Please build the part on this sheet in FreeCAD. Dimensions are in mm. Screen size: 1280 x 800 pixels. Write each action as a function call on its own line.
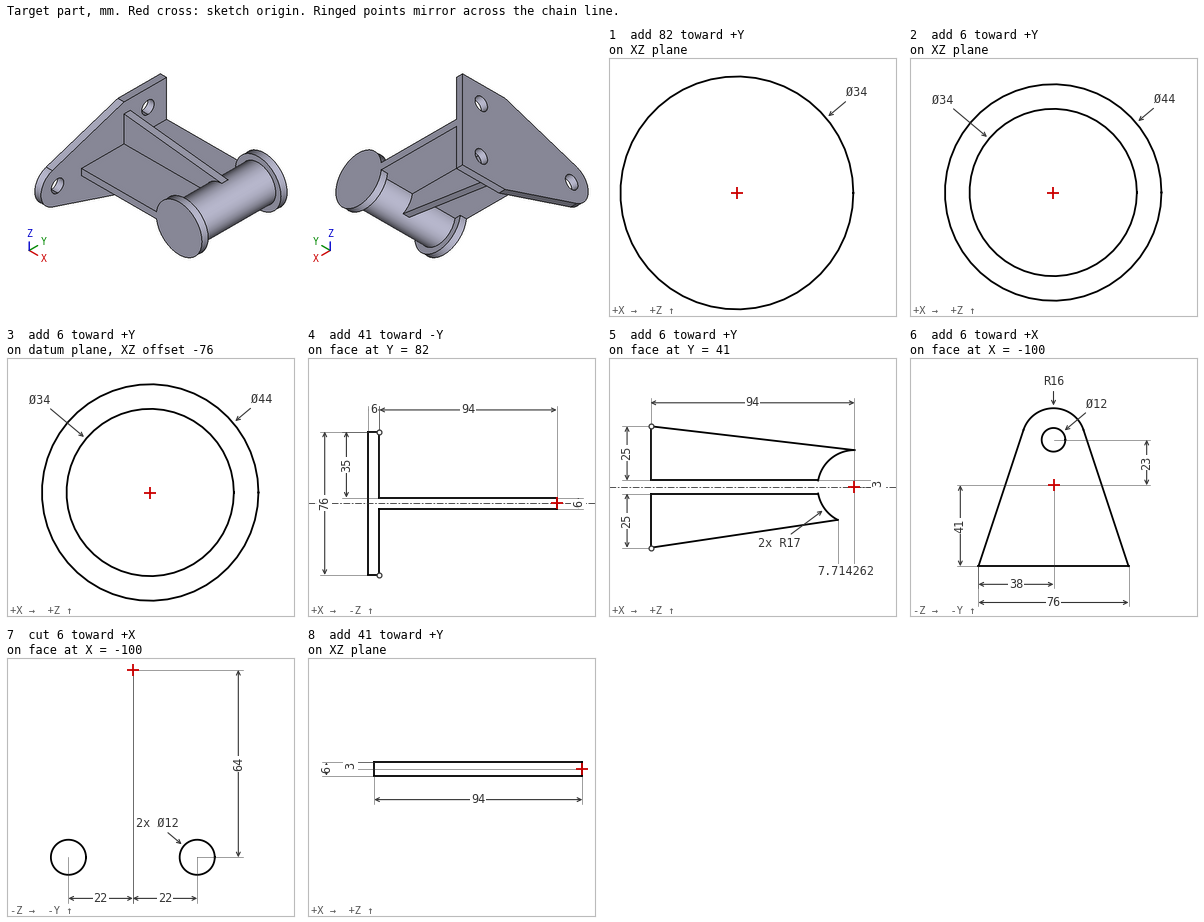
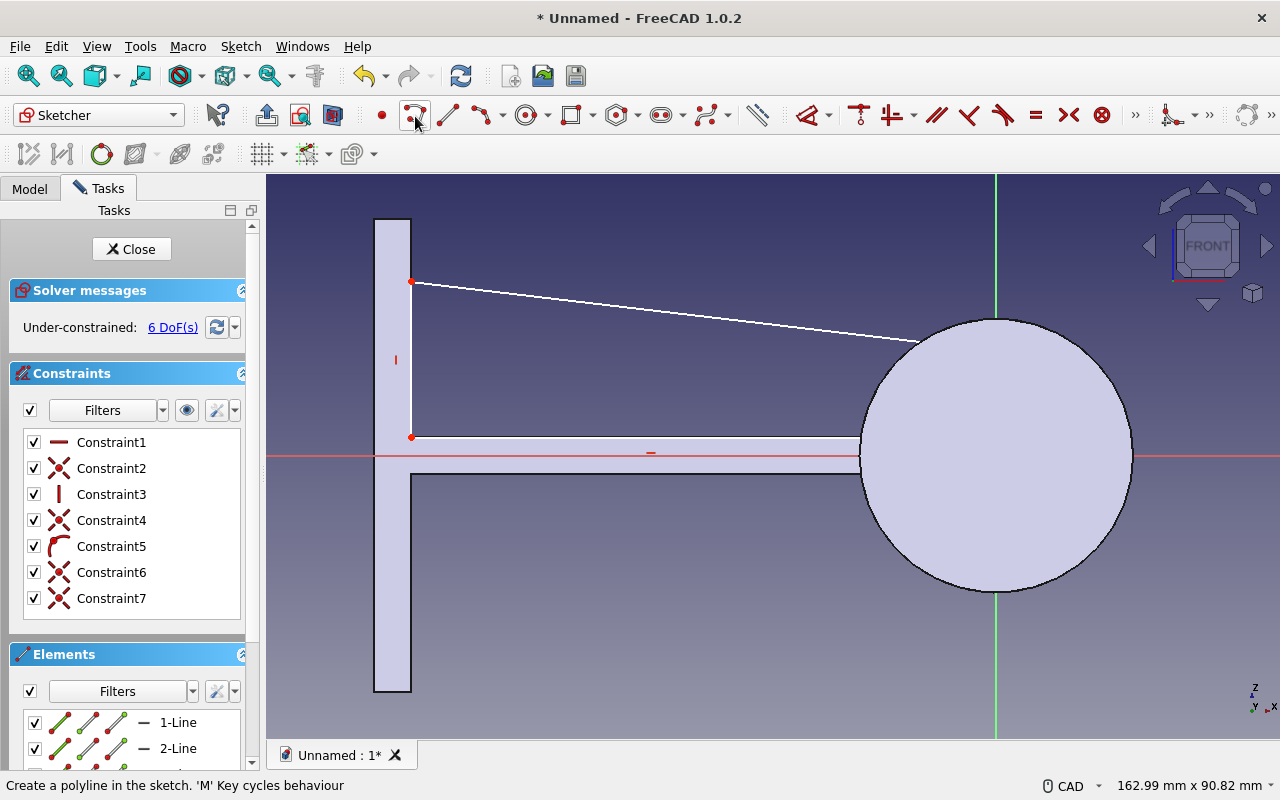
click(948, 550)
click(411, 630)
click(411, 474)
click(892, 474)
right_click(892, 474)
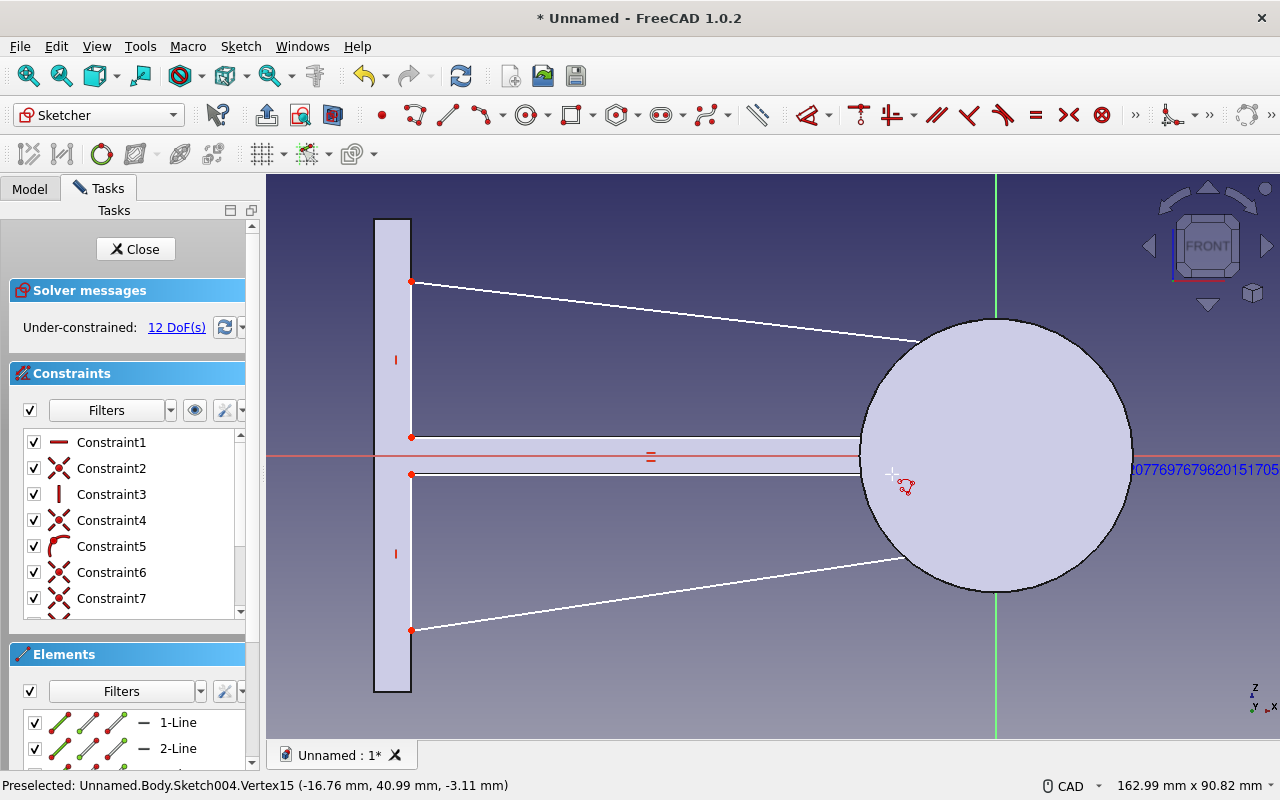
click(480, 116)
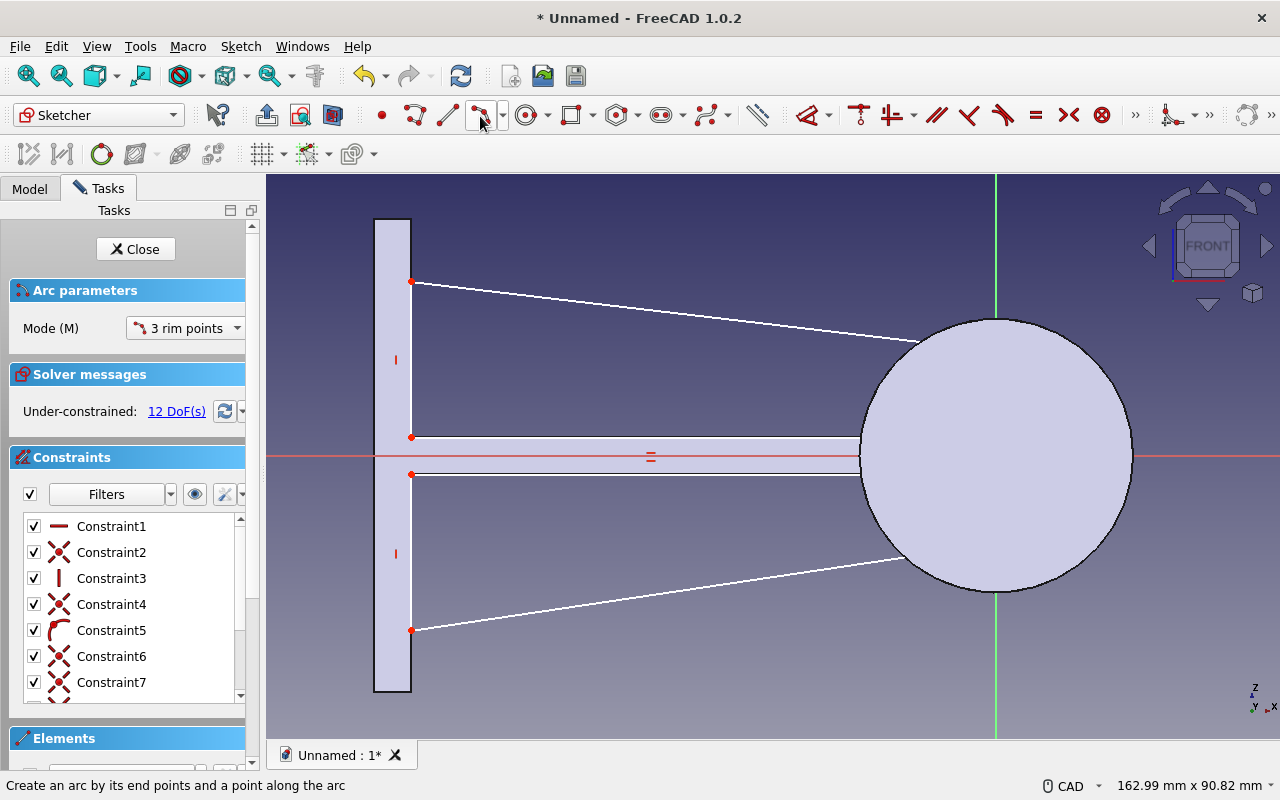
click(892, 475)
click(948, 551)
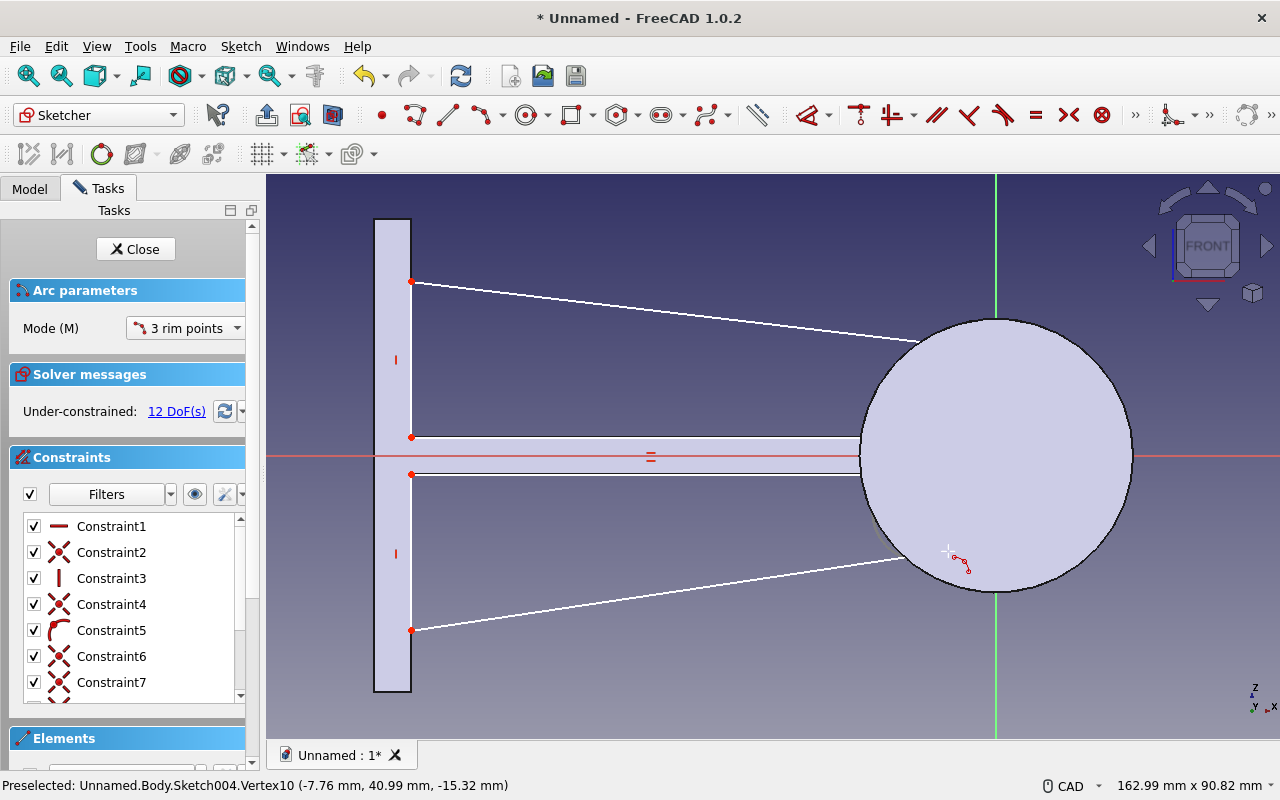
scroll(911, 519, up, 2)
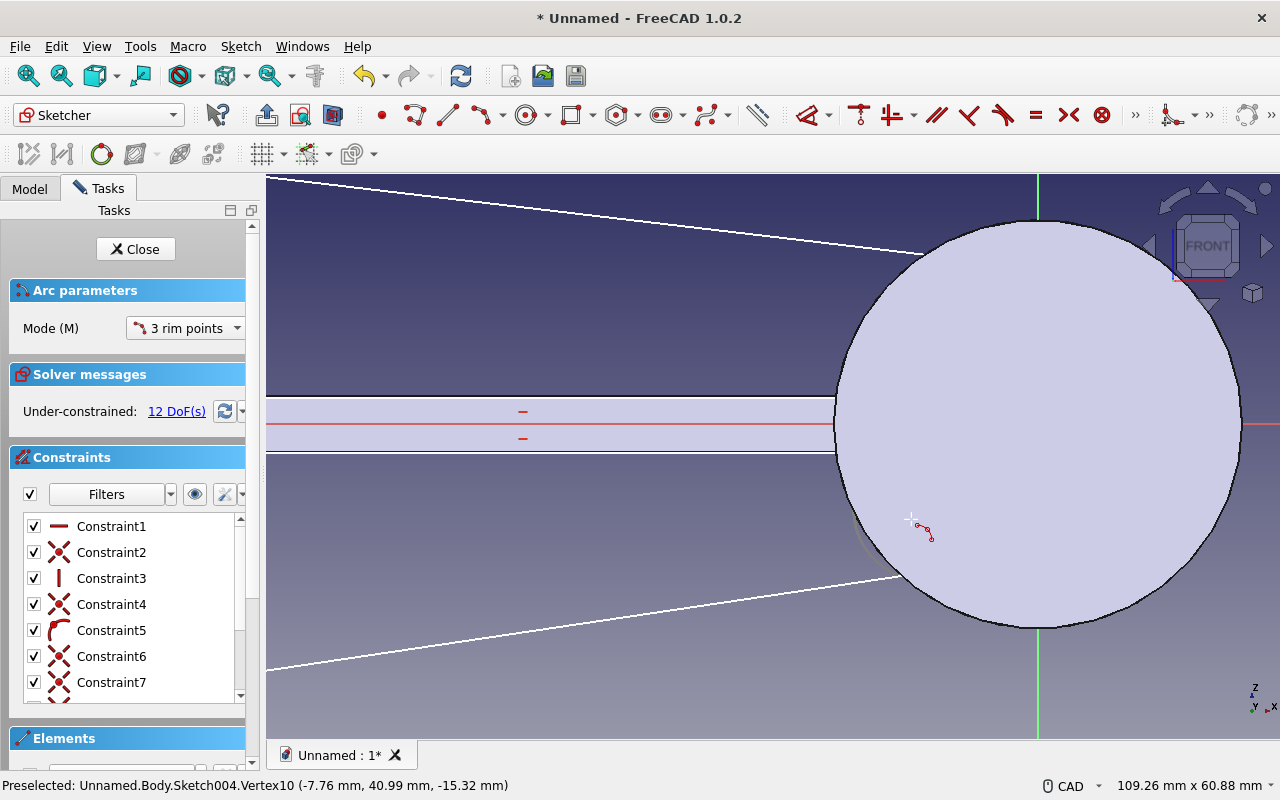
click(911, 518)
key(Escape)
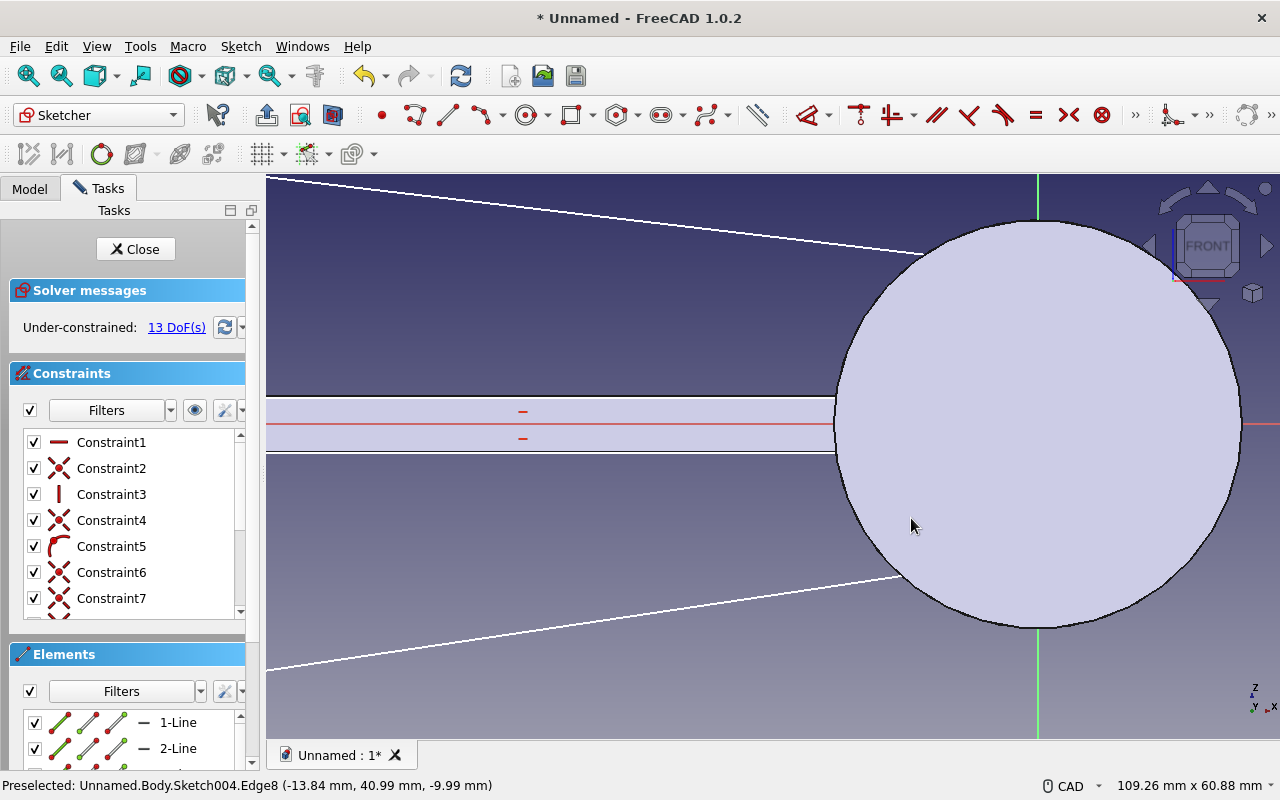
click(974, 282)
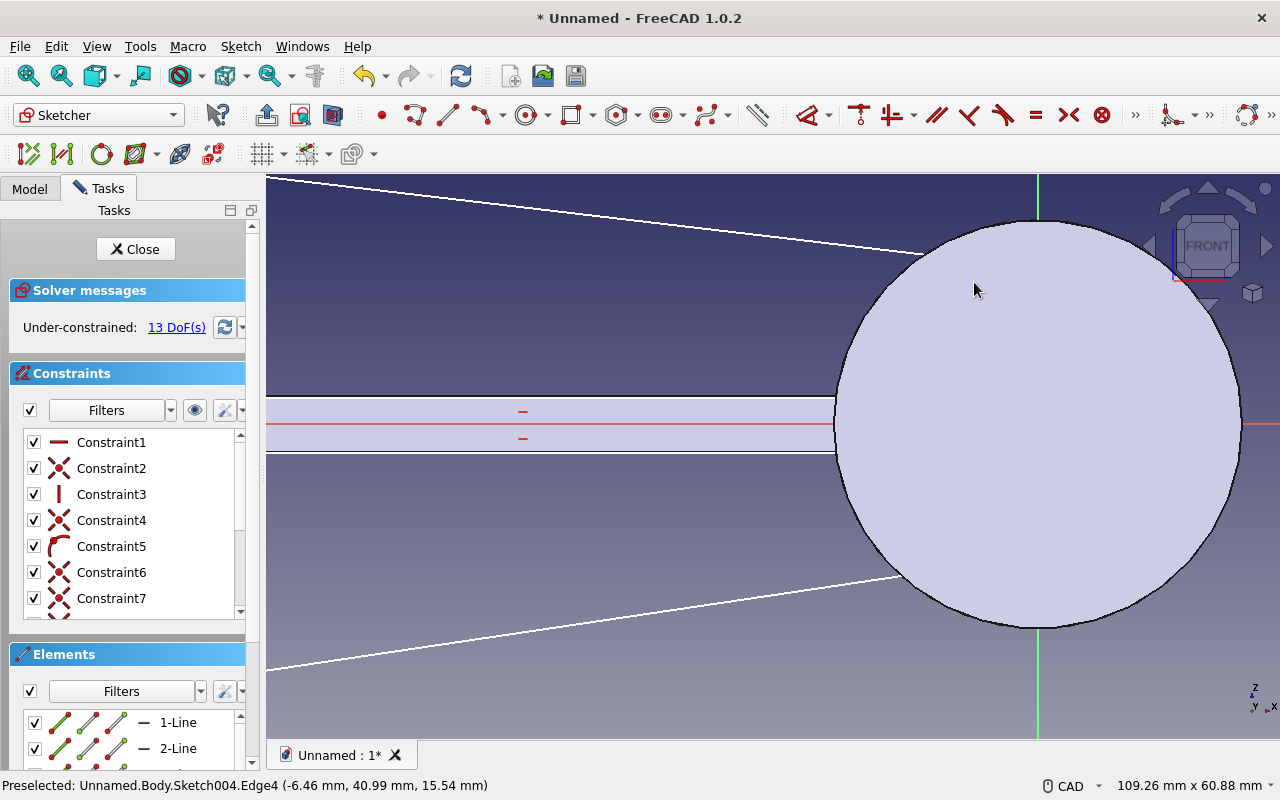
click(896, 494)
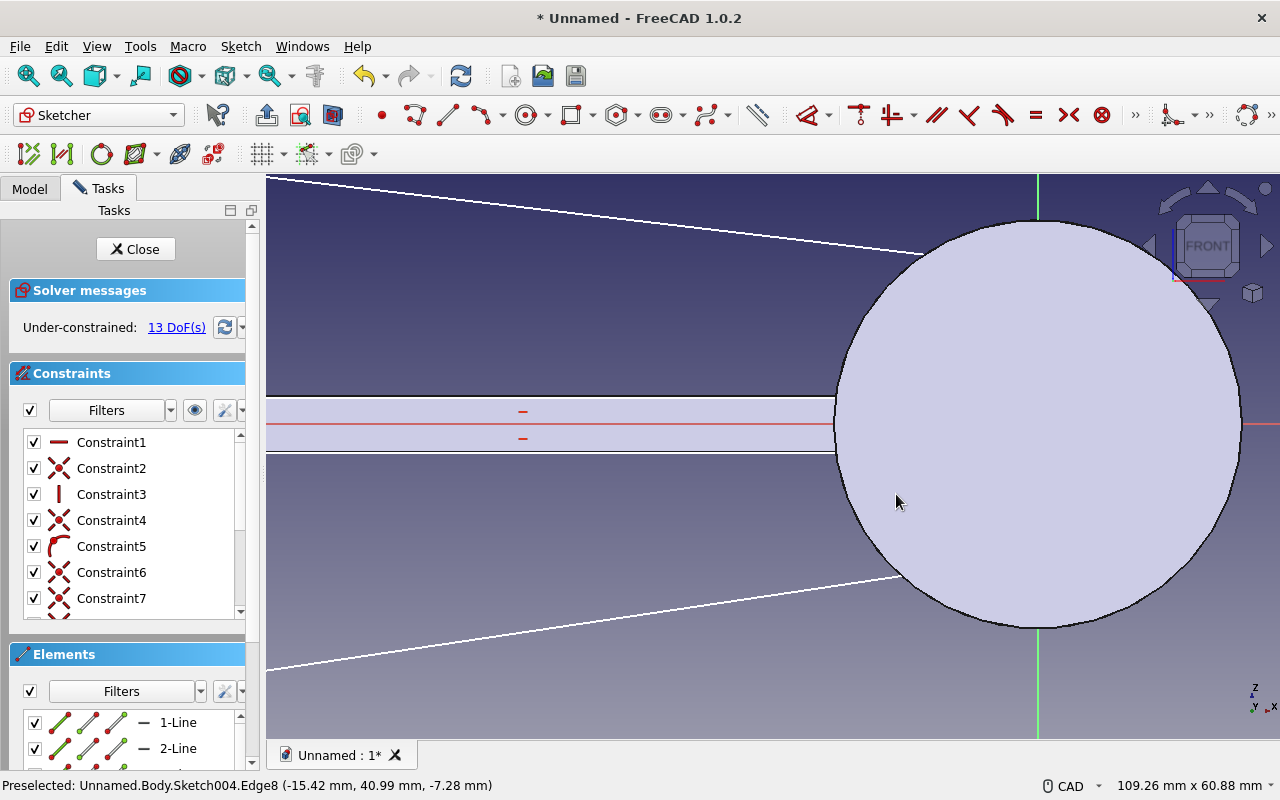
key(c)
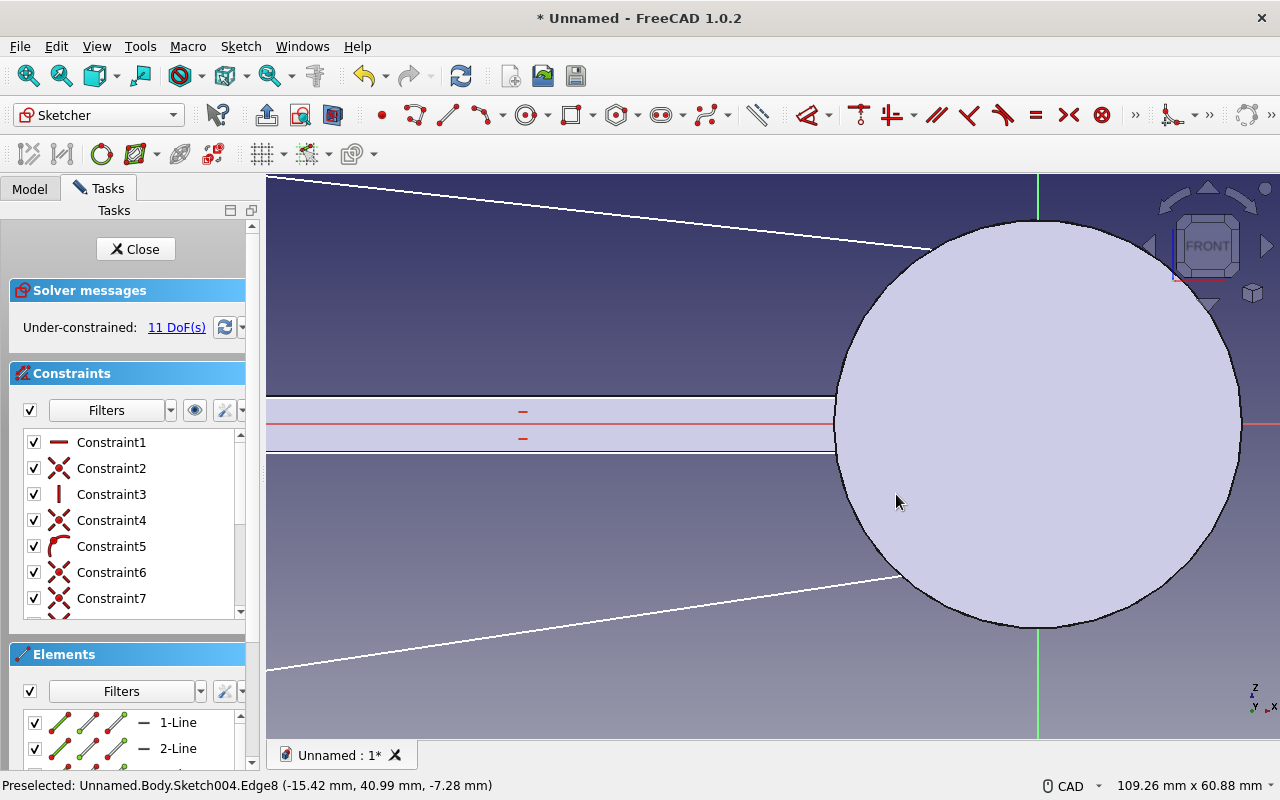
drag(1028, 413, 1052, 434)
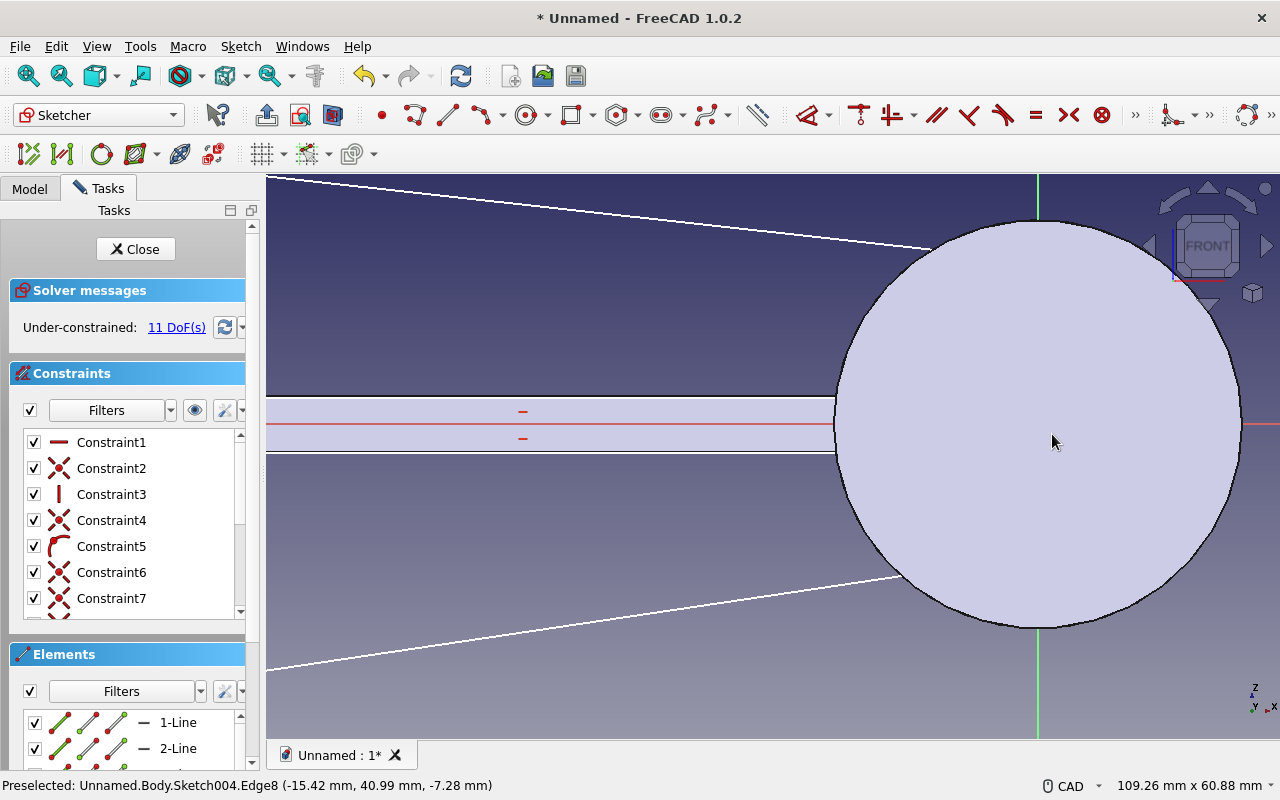
click(859, 116)